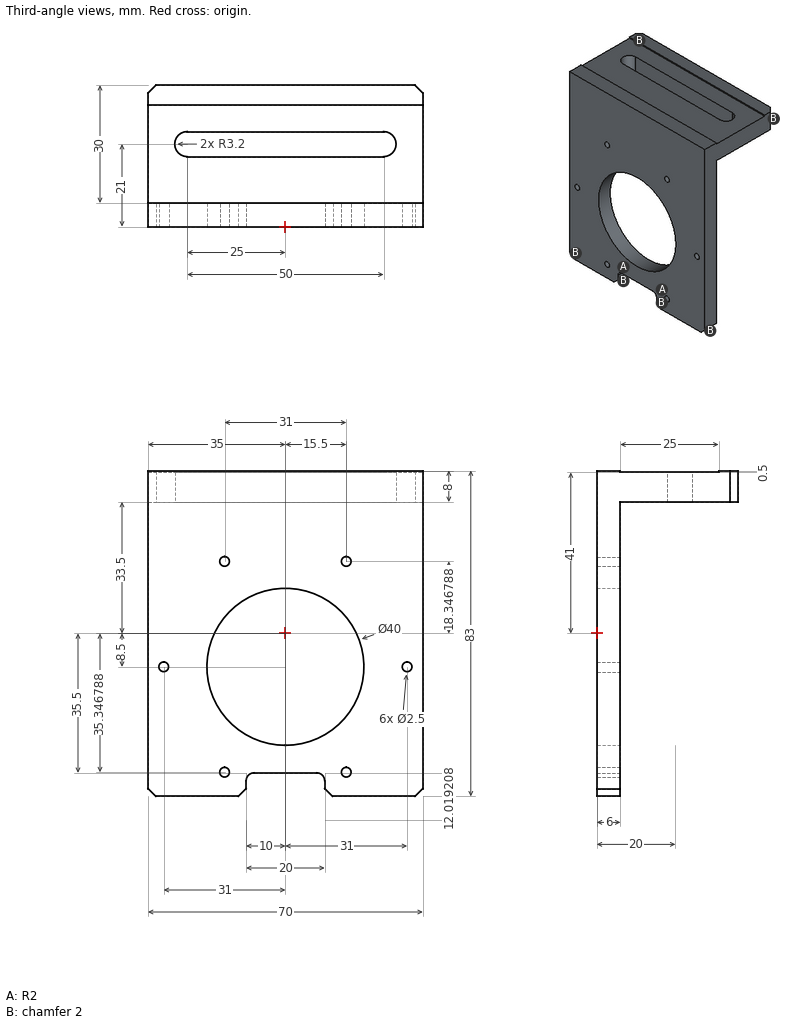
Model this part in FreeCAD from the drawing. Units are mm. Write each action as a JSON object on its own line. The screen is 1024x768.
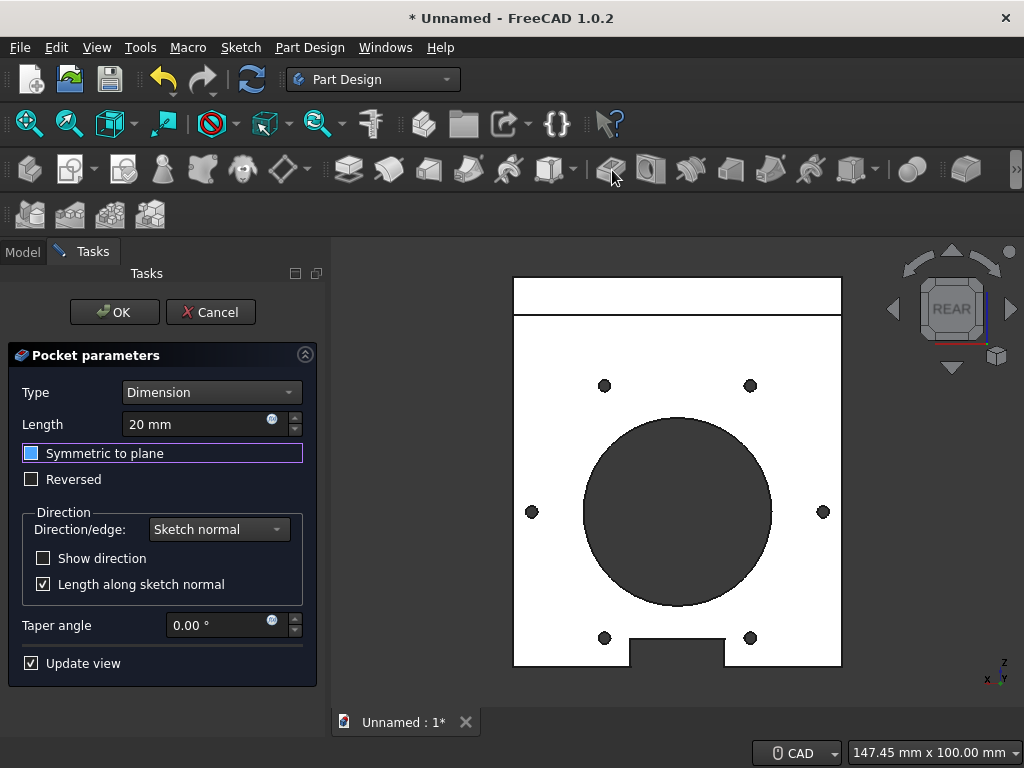
{"action": "left_click", "coordinate": [115, 312]}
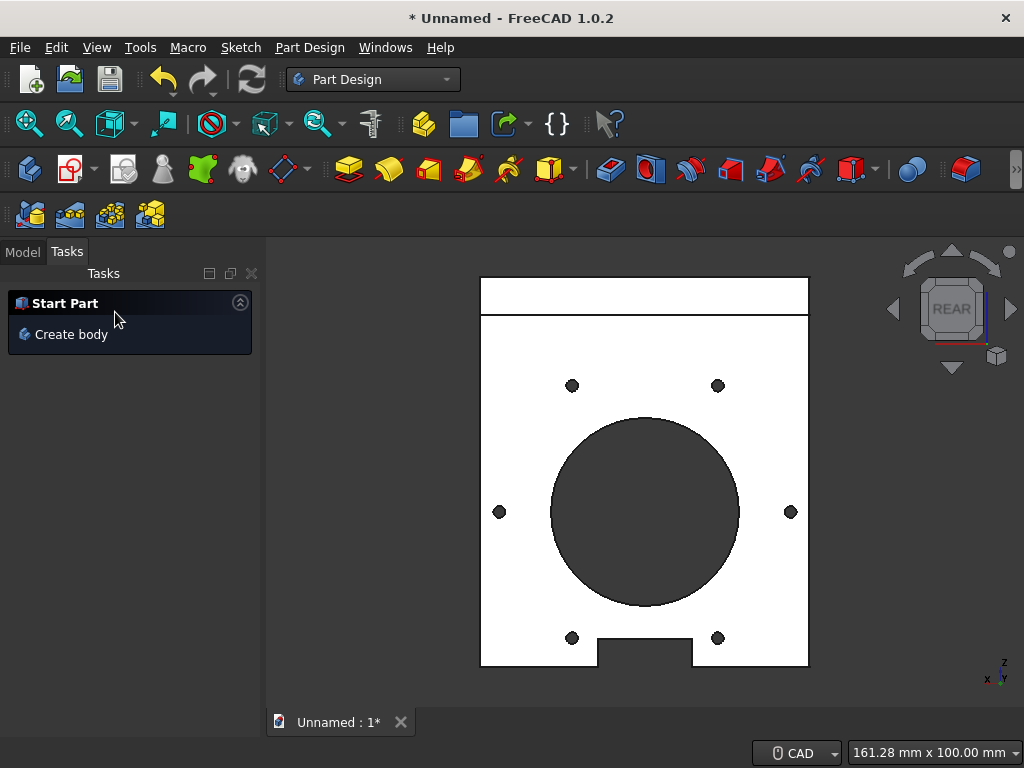
{"action": "key", "text": "5"}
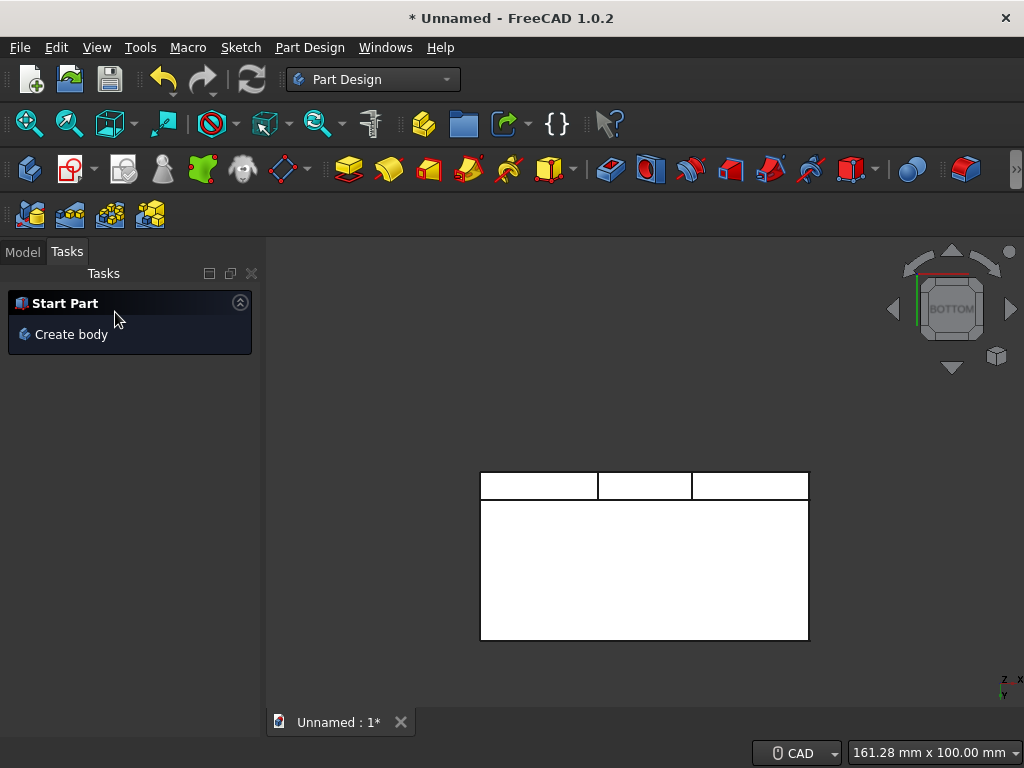
{"action": "left_click", "coordinate": [30, 124]}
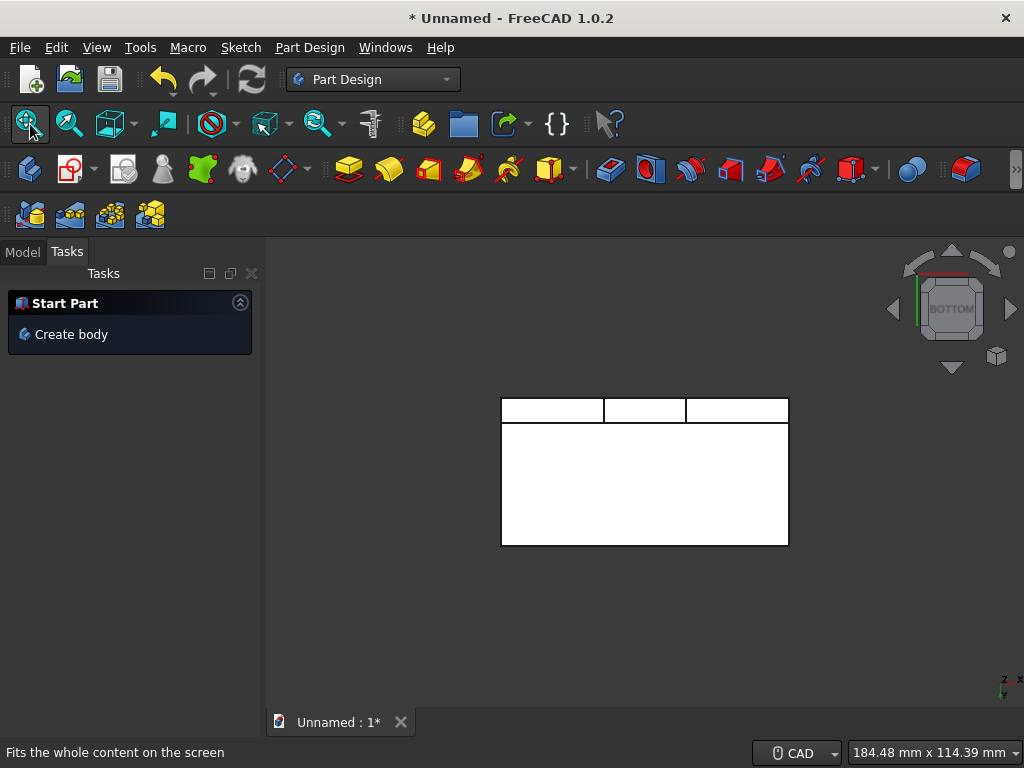
{"action": "left_click", "coordinate": [727, 483]}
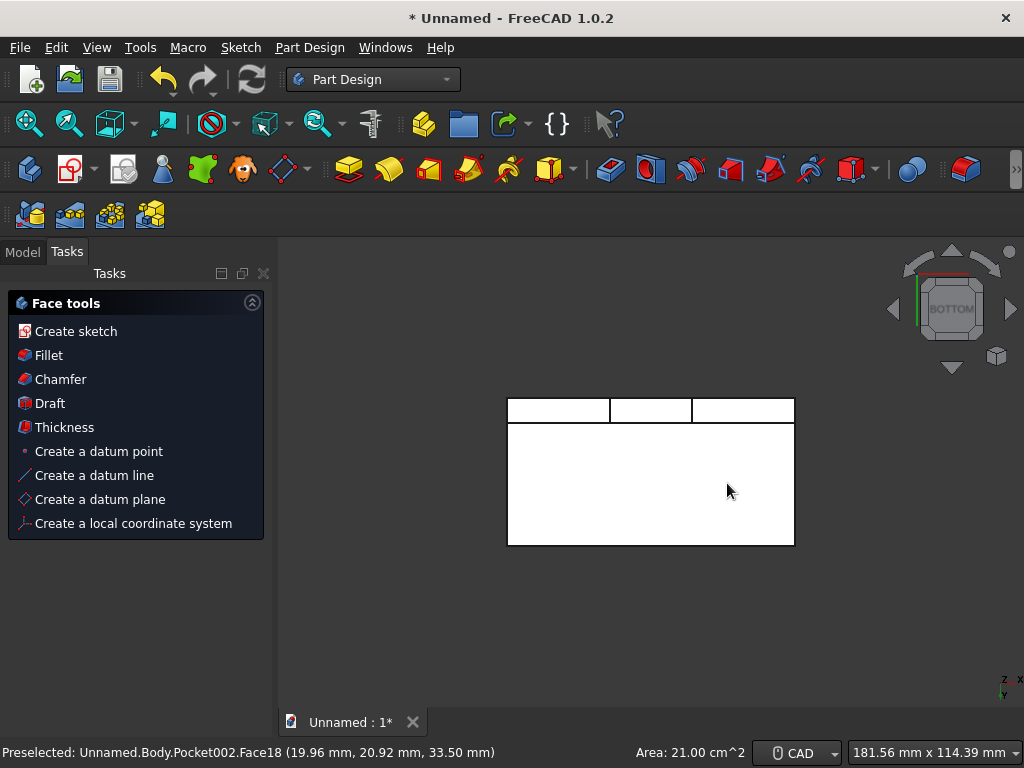
{"action": "left_click", "coordinate": [70, 170]}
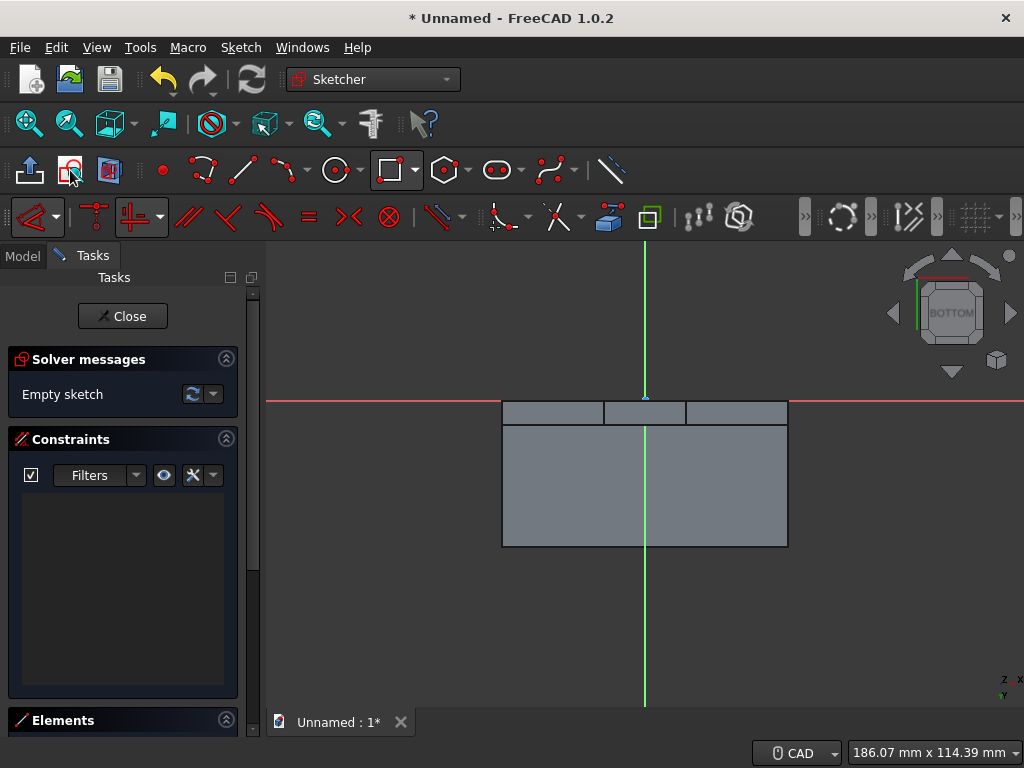
{"action": "left_click", "coordinate": [110, 170]}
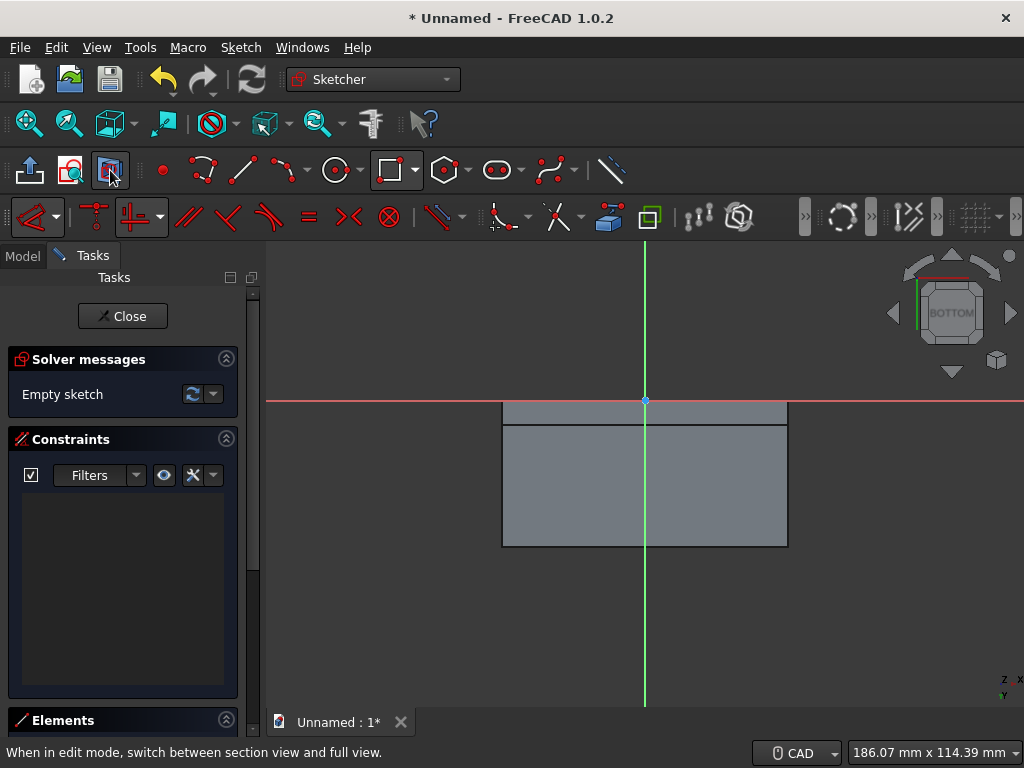
{"action": "scroll", "coordinate": [728, 421], "scroll_direction": "up", "scroll_amount": 3}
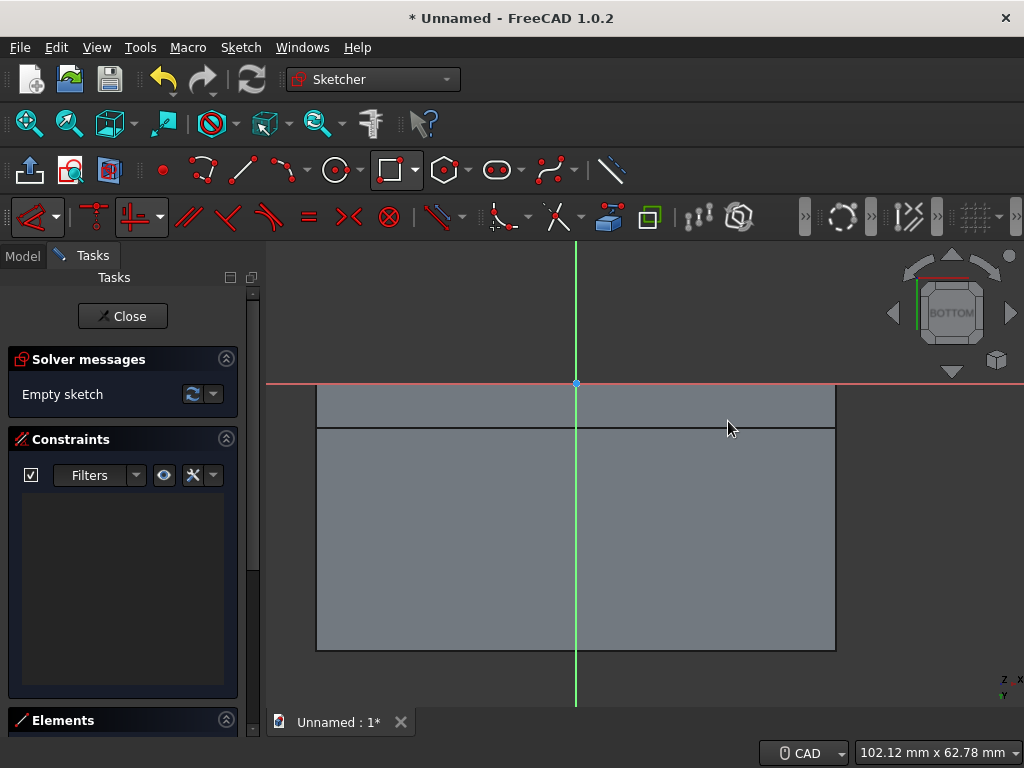
{"action": "left_click", "coordinate": [498, 170]}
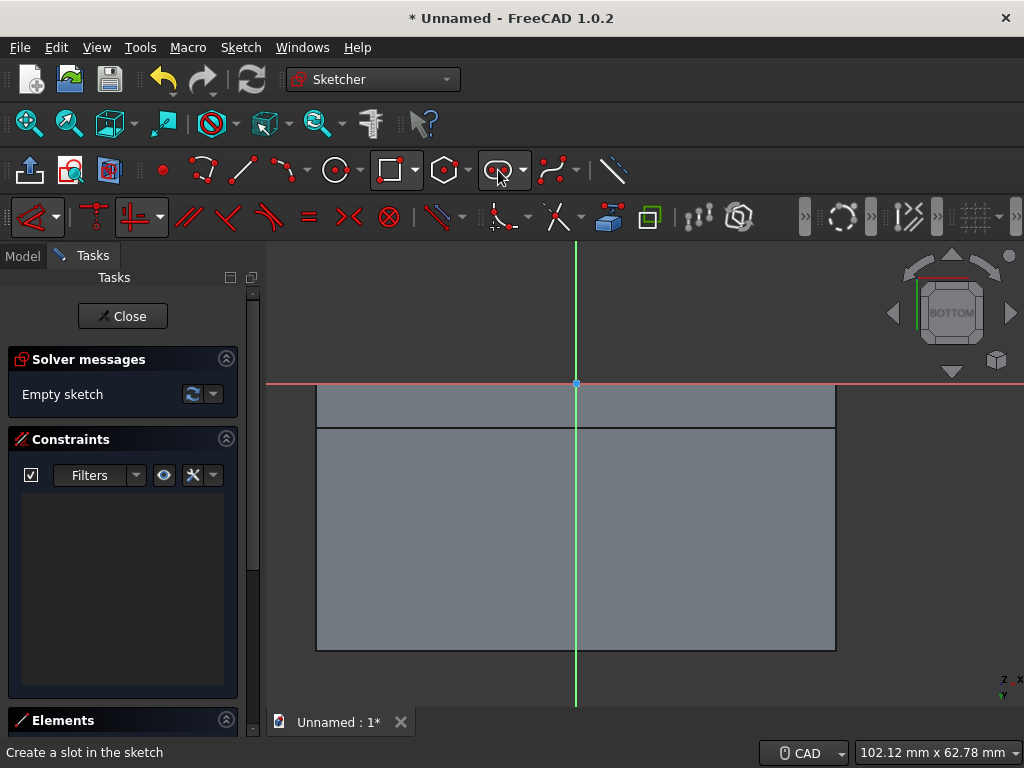
{"action": "left_click", "coordinate": [391, 540]}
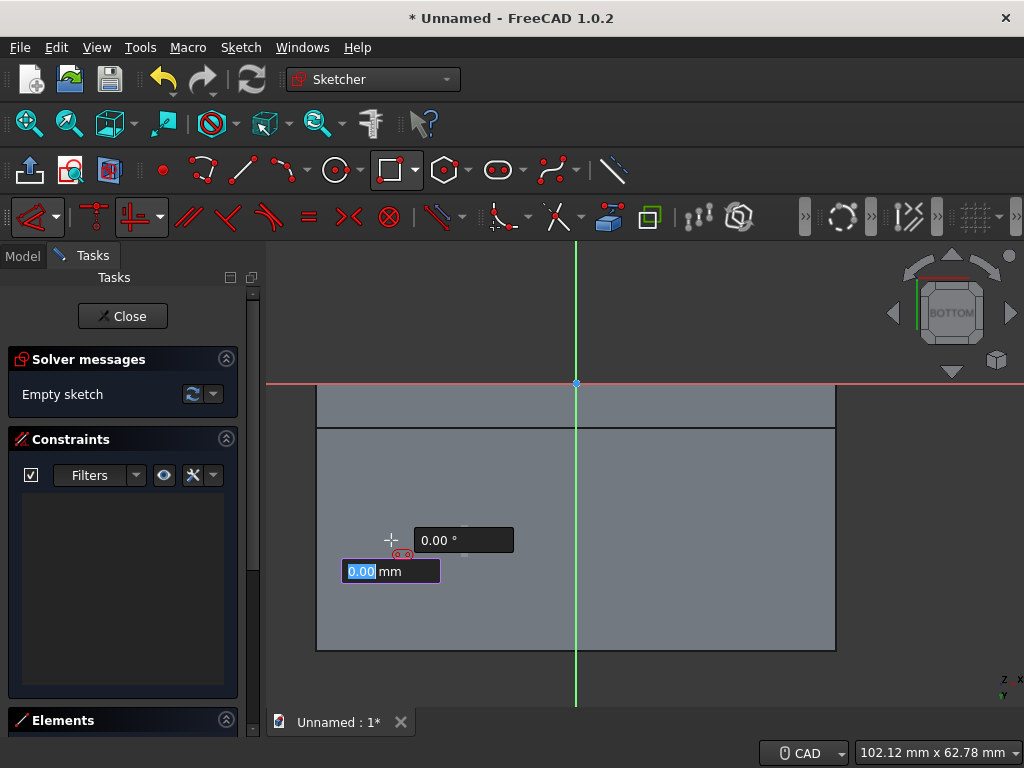
{"action": "left_click", "coordinate": [762, 540]}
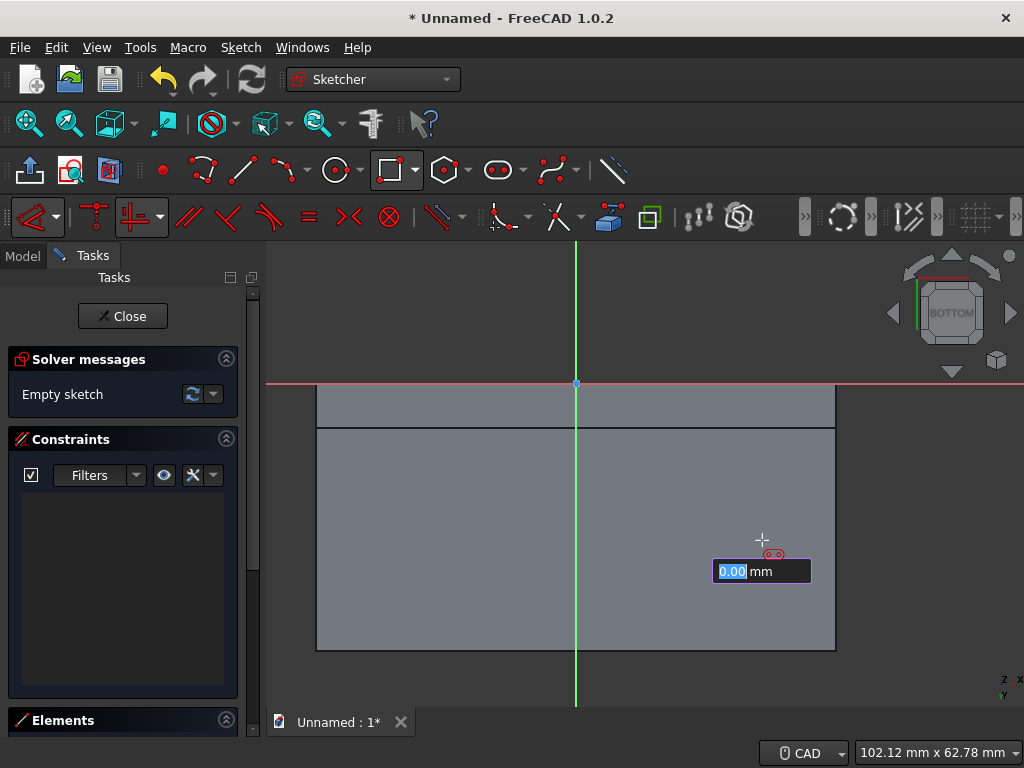
{"action": "left_click", "coordinate": [632, 516]}
{"action": "key", "text": "Escape"}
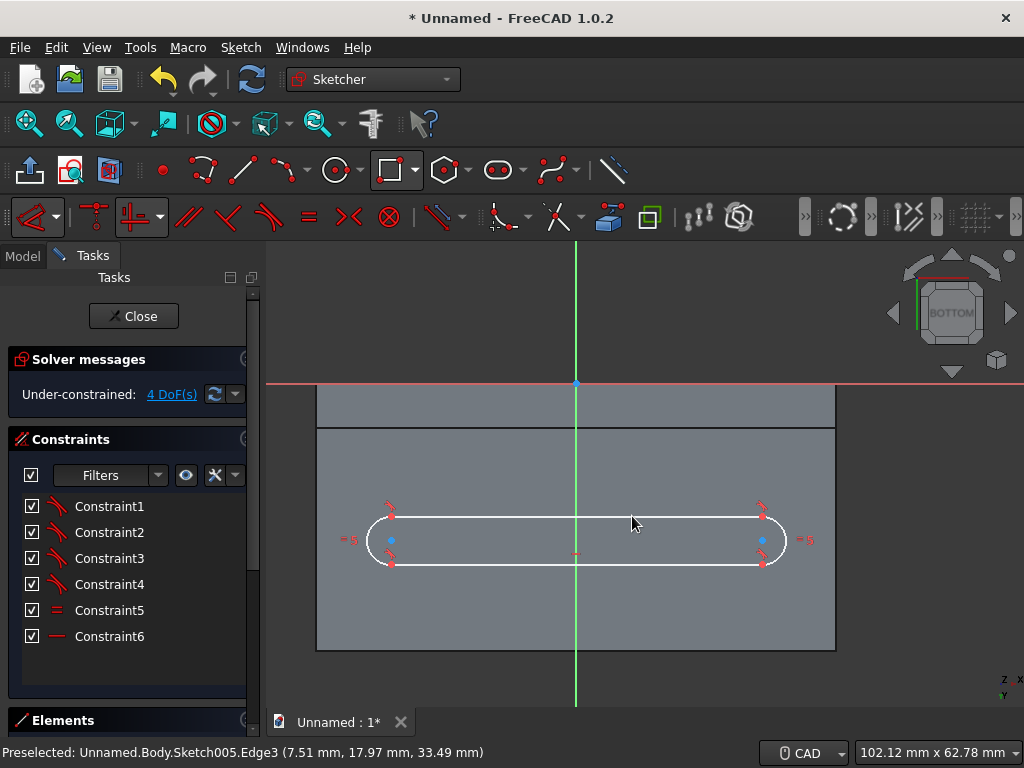
{"action": "scroll", "coordinate": [372, 527], "scroll_direction": "up", "scroll_amount": 3}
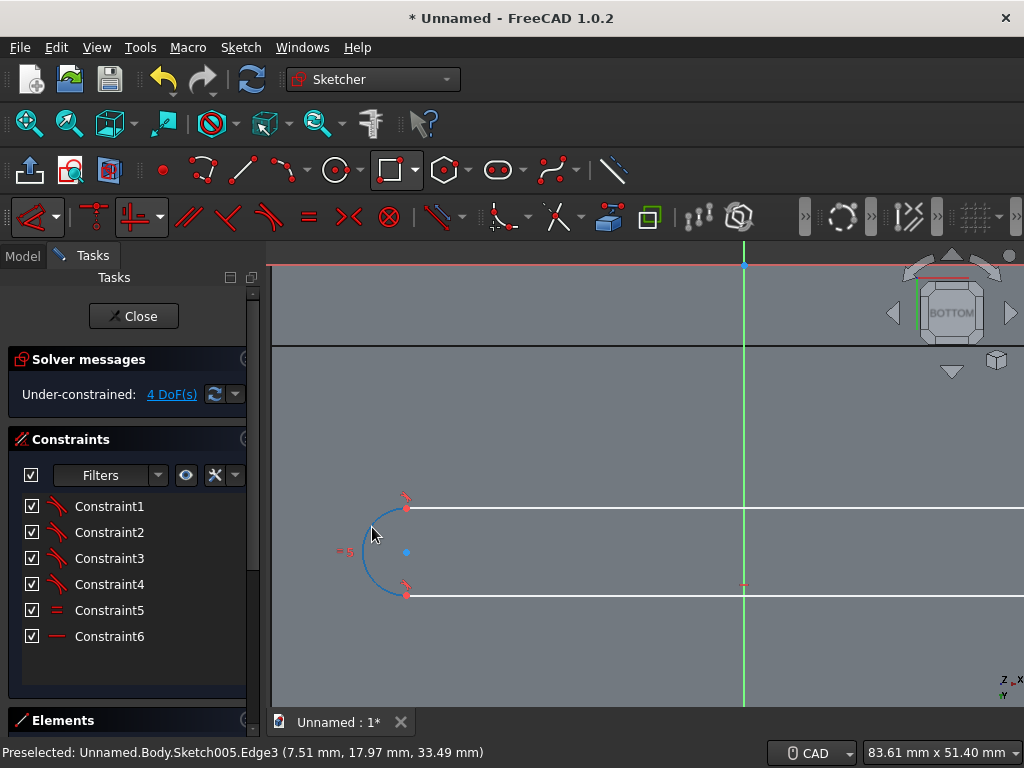
{"action": "left_click", "coordinate": [371, 526]}